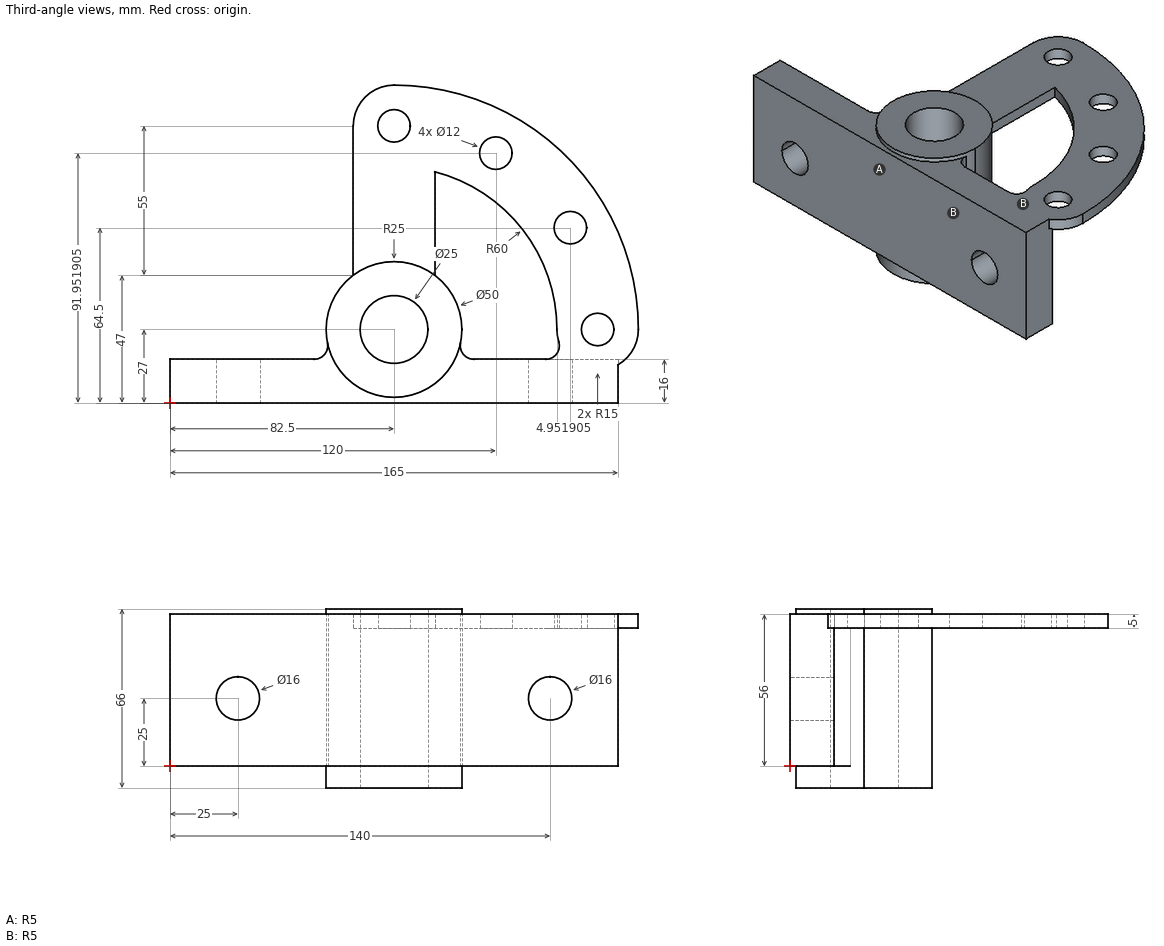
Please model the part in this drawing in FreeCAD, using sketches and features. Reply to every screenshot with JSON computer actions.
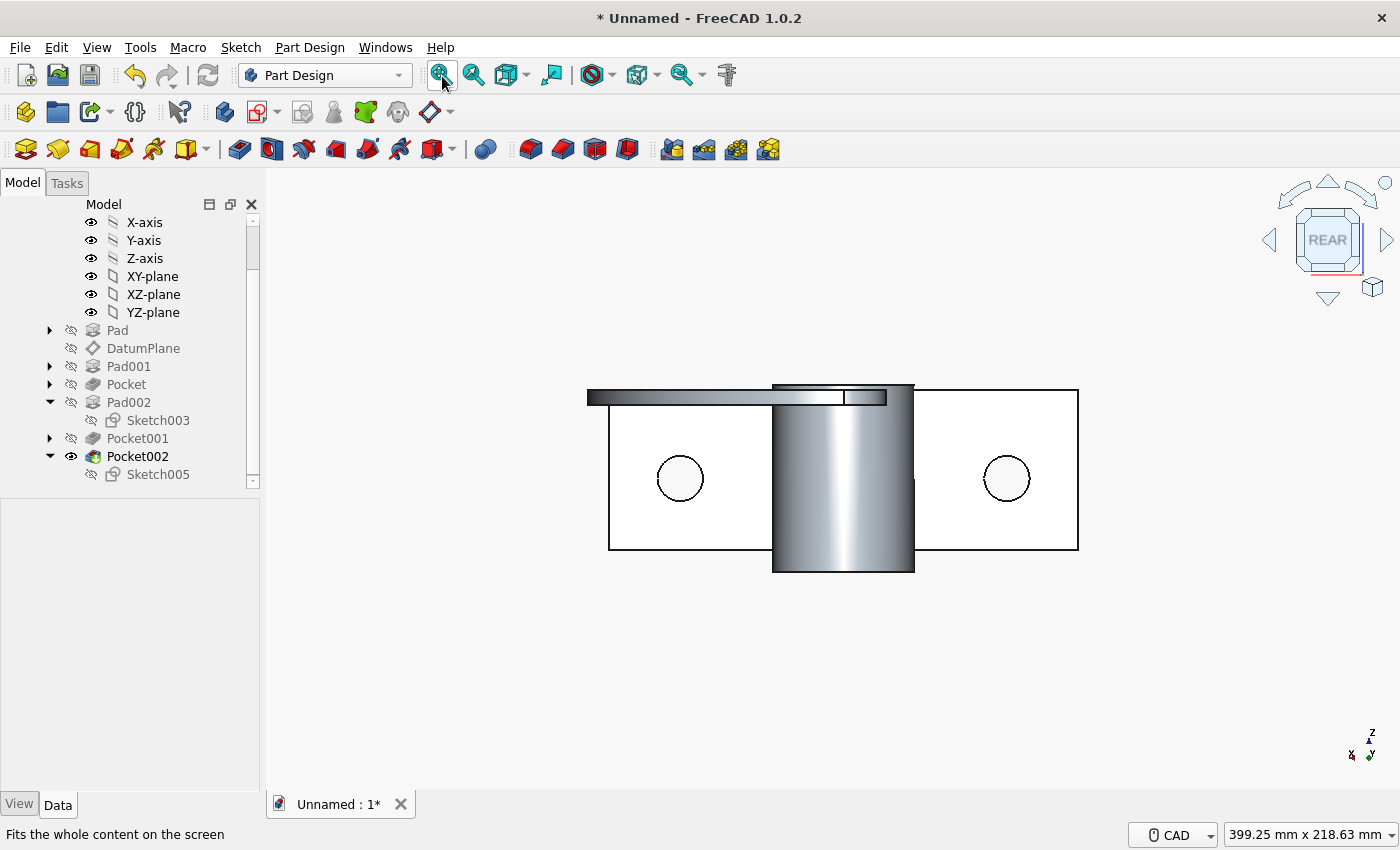
{"action": "left_click", "coordinate": [442, 76]}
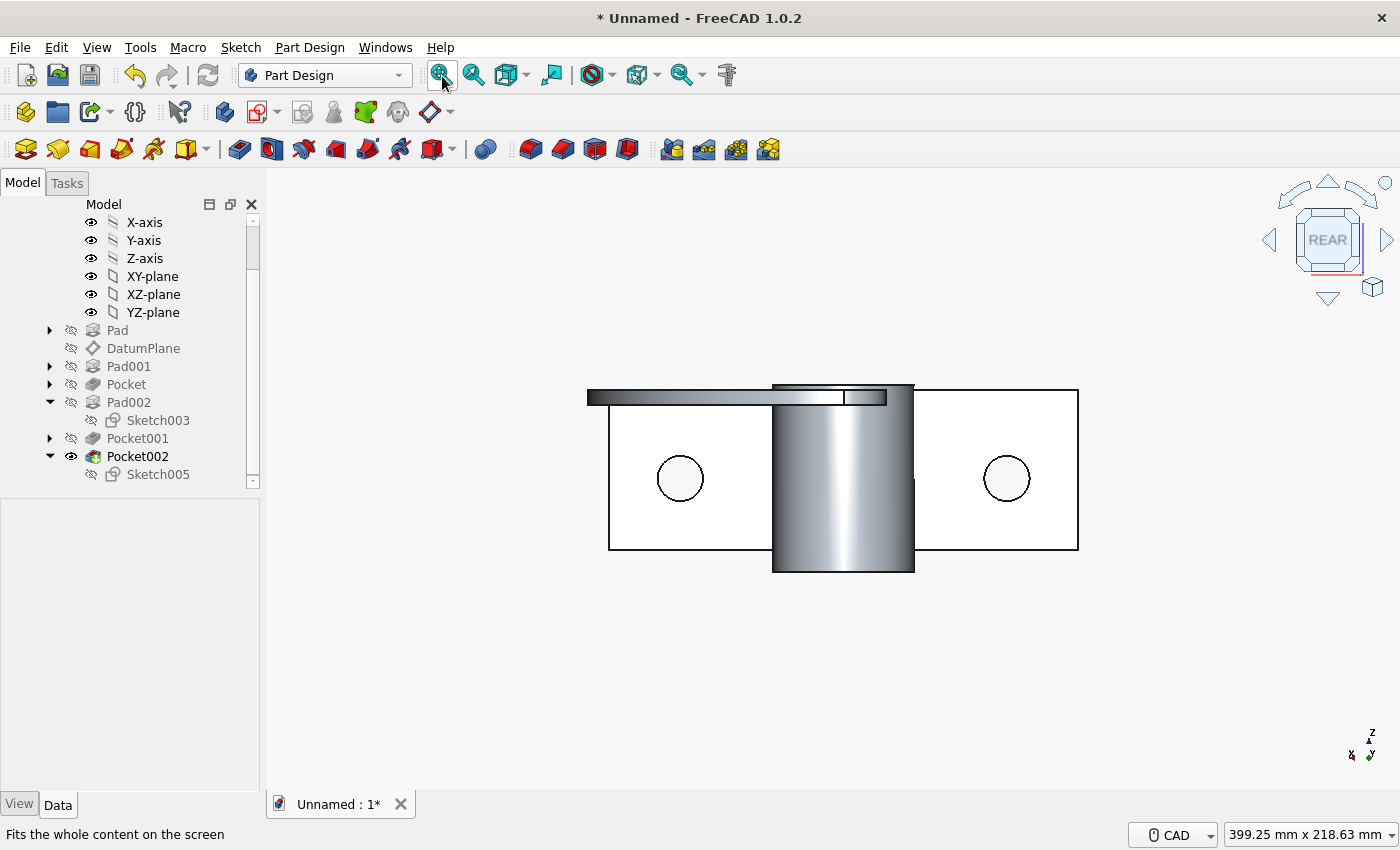
{"action": "key", "text": "6"}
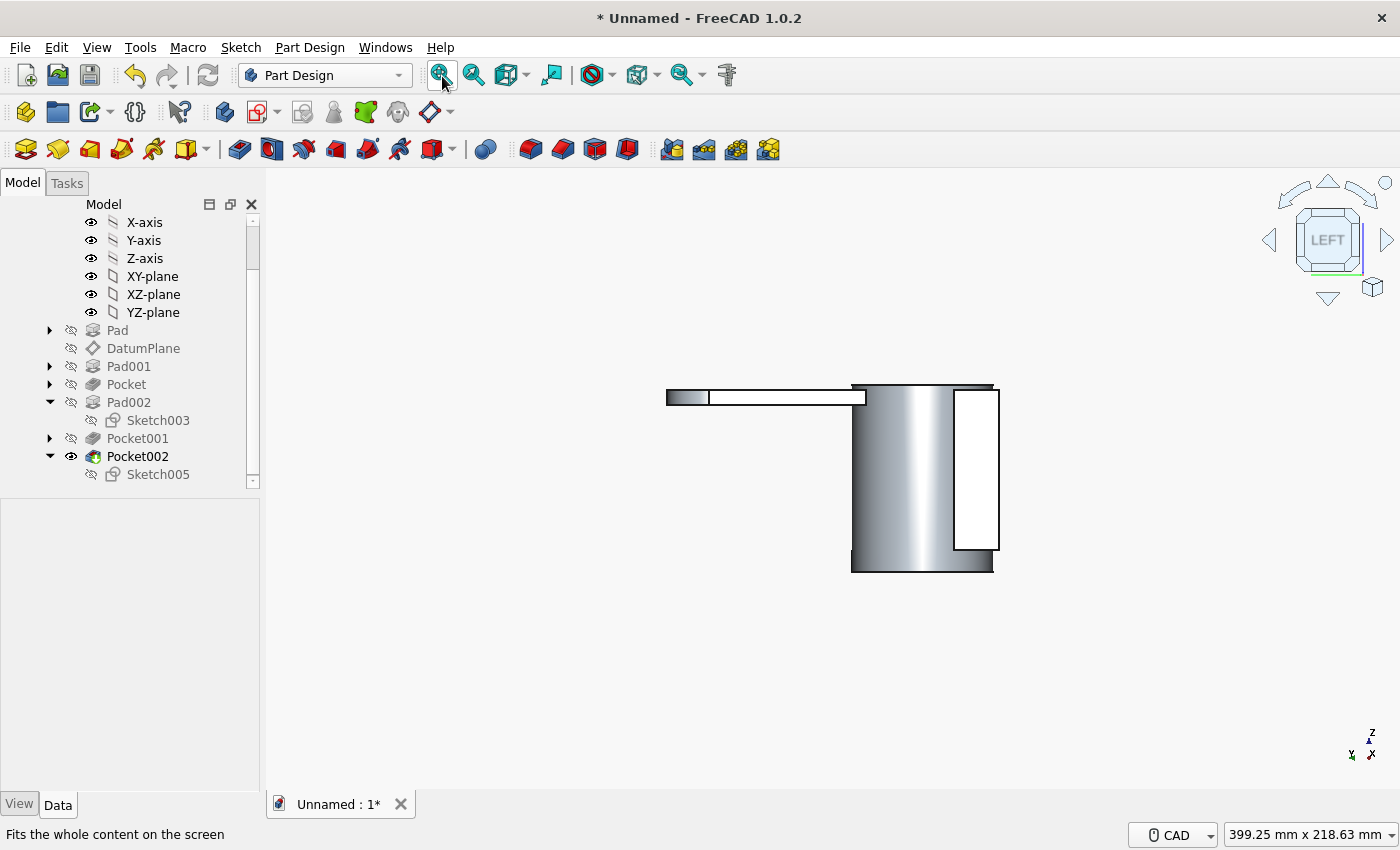
{"action": "left_click", "coordinate": [442, 76]}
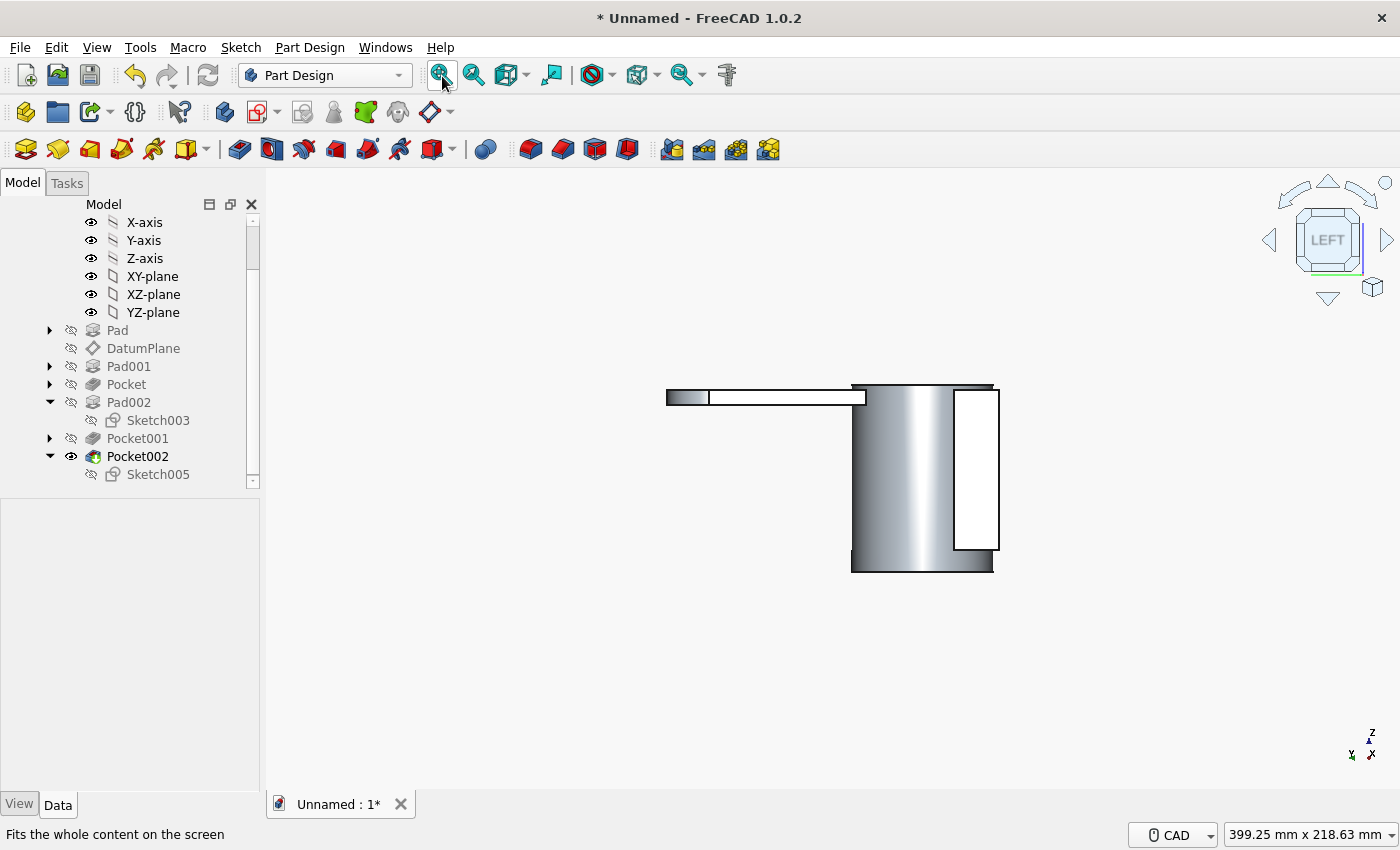
{"action": "key", "text": "v 3"}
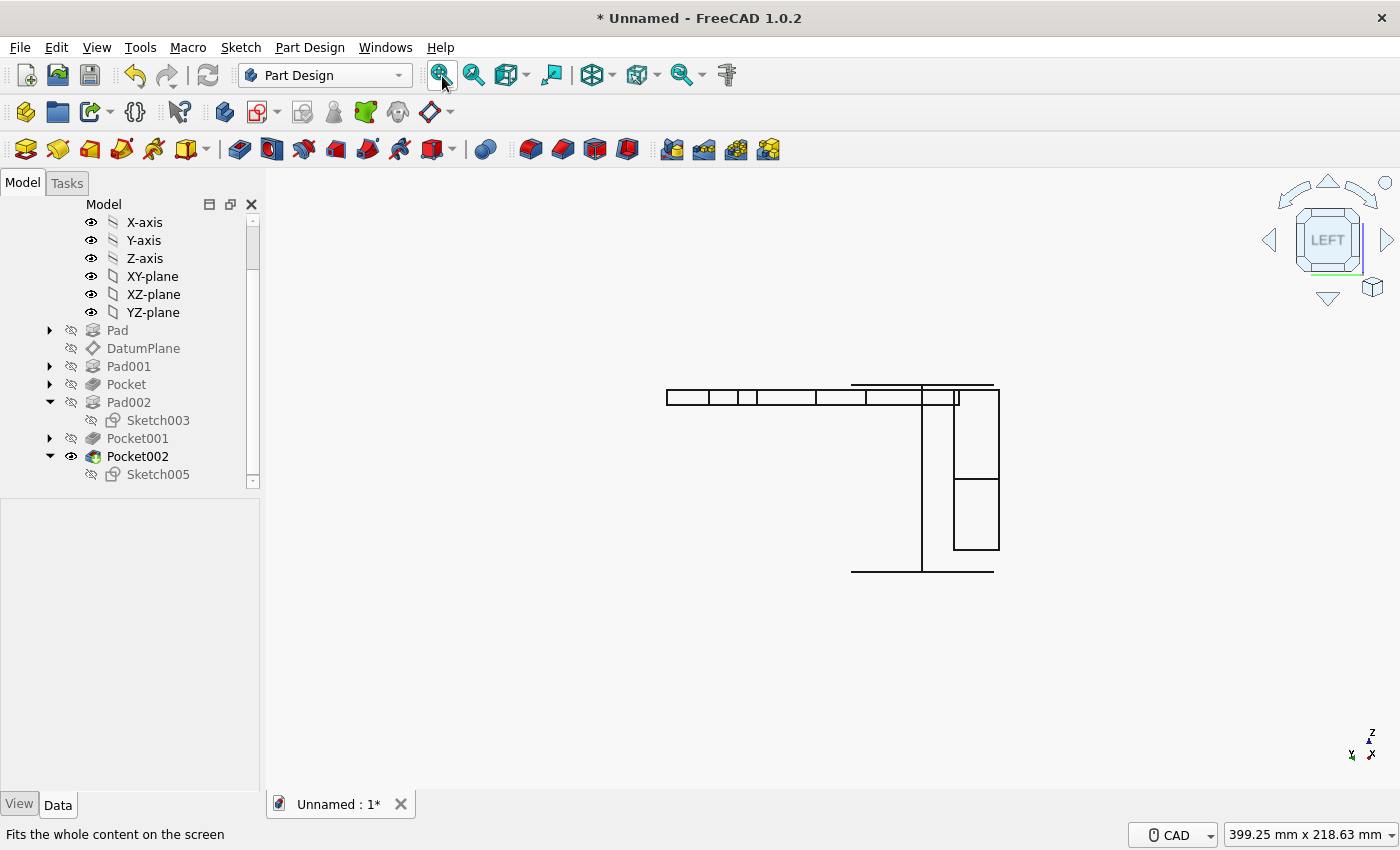
{"action": "key", "text": "0"}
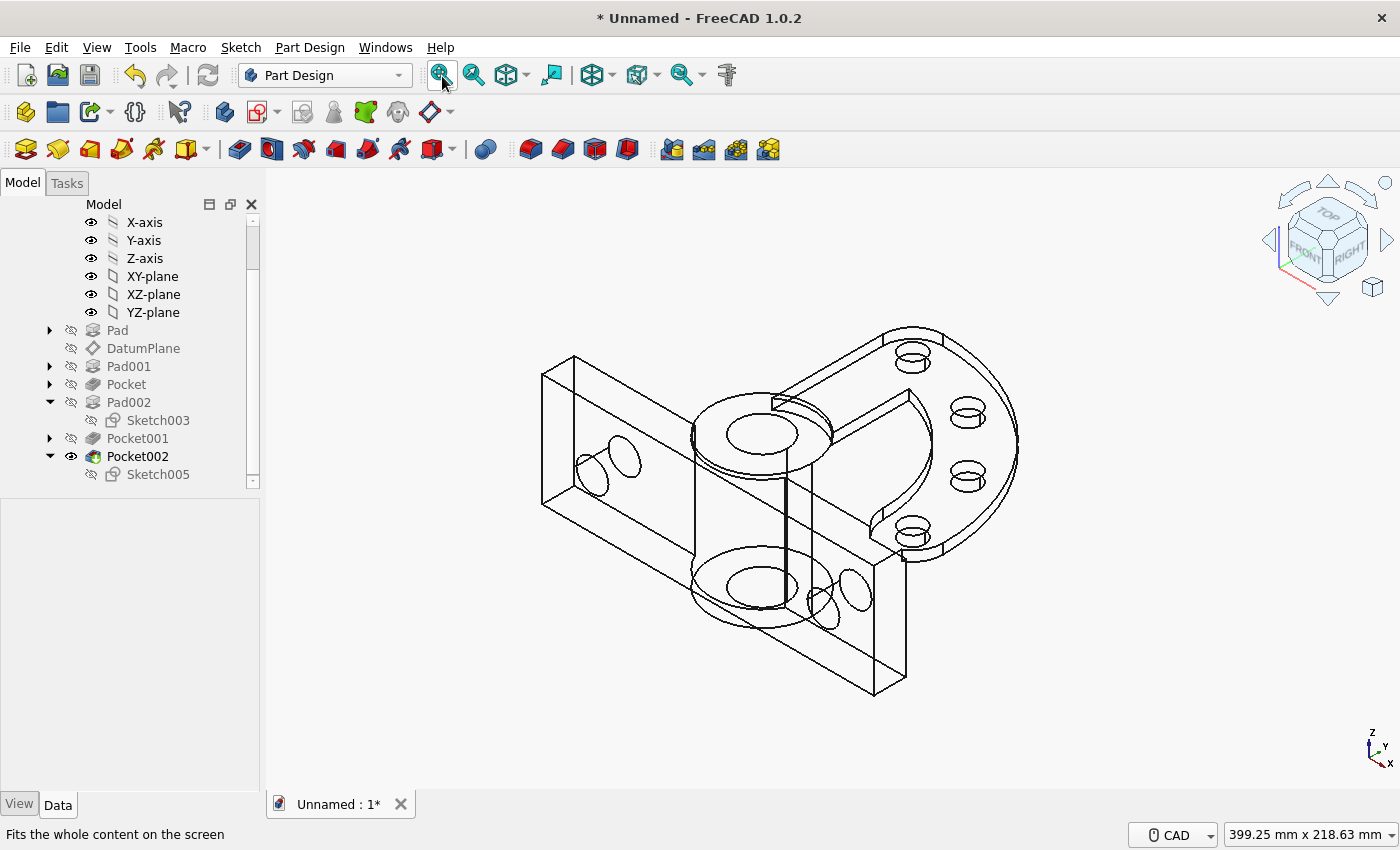
{"action": "left_click", "coordinate": [695, 489]}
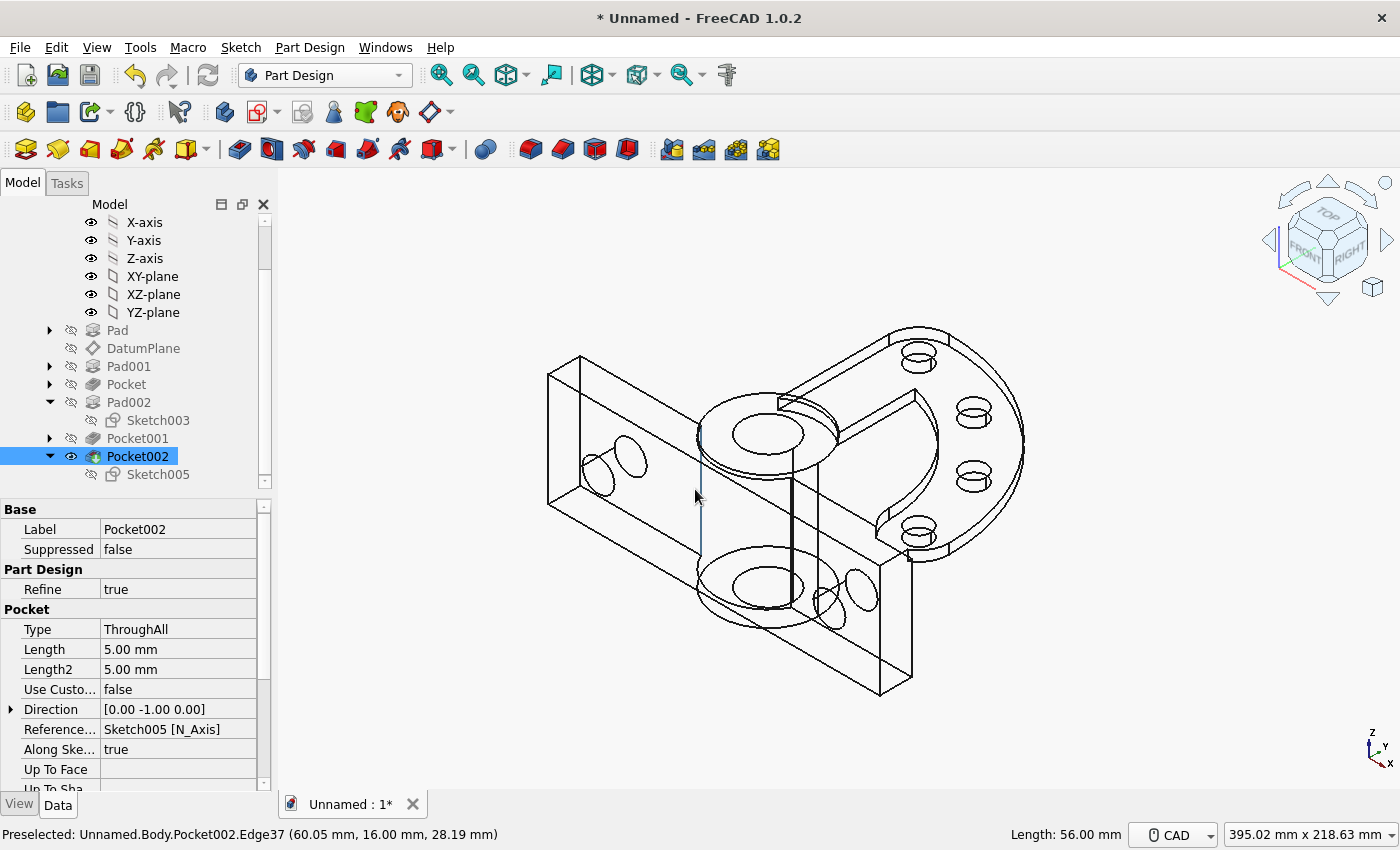
{"action": "key", "text": "v 1"}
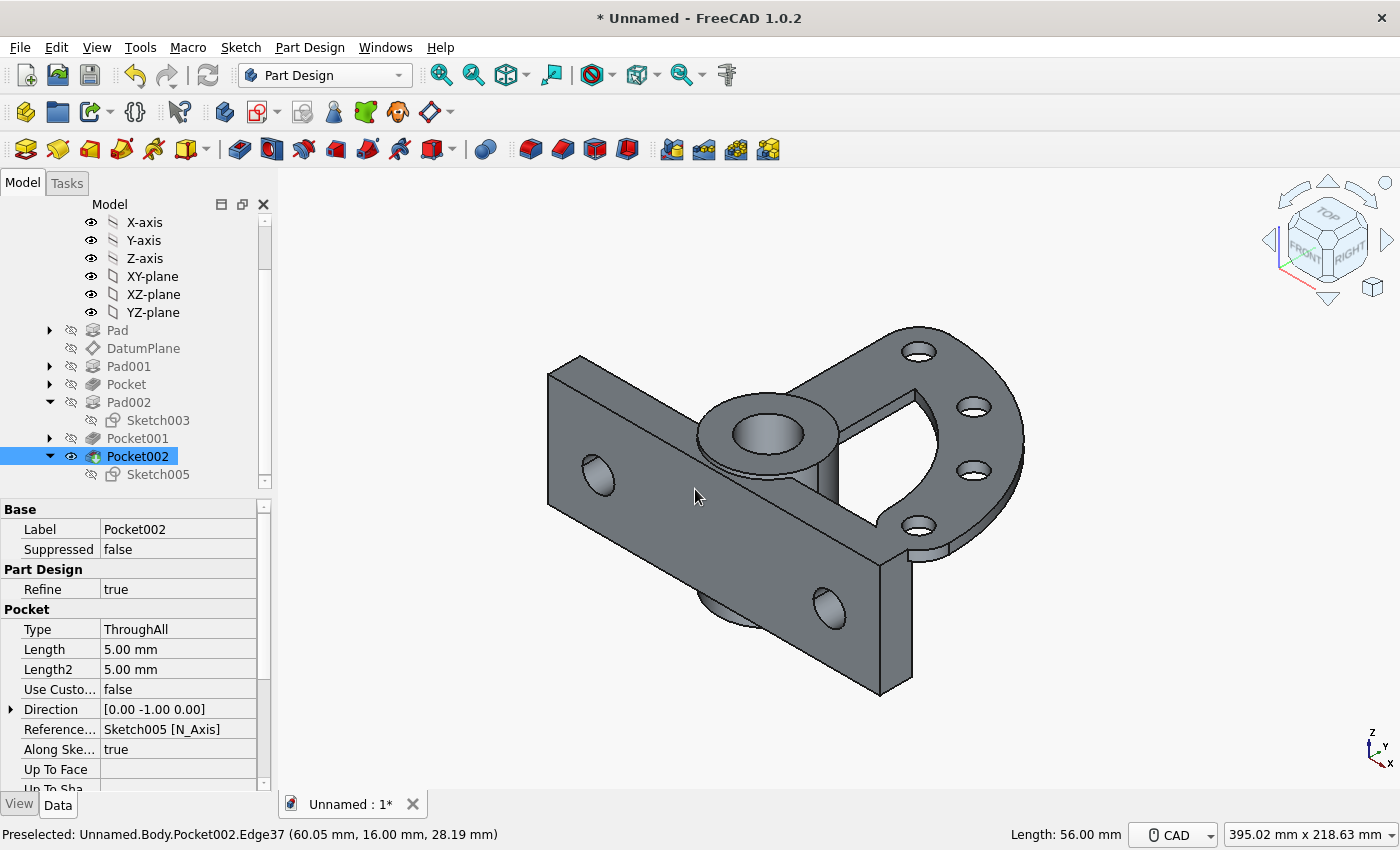
{"action": "left_click", "coordinate": [532, 150]}